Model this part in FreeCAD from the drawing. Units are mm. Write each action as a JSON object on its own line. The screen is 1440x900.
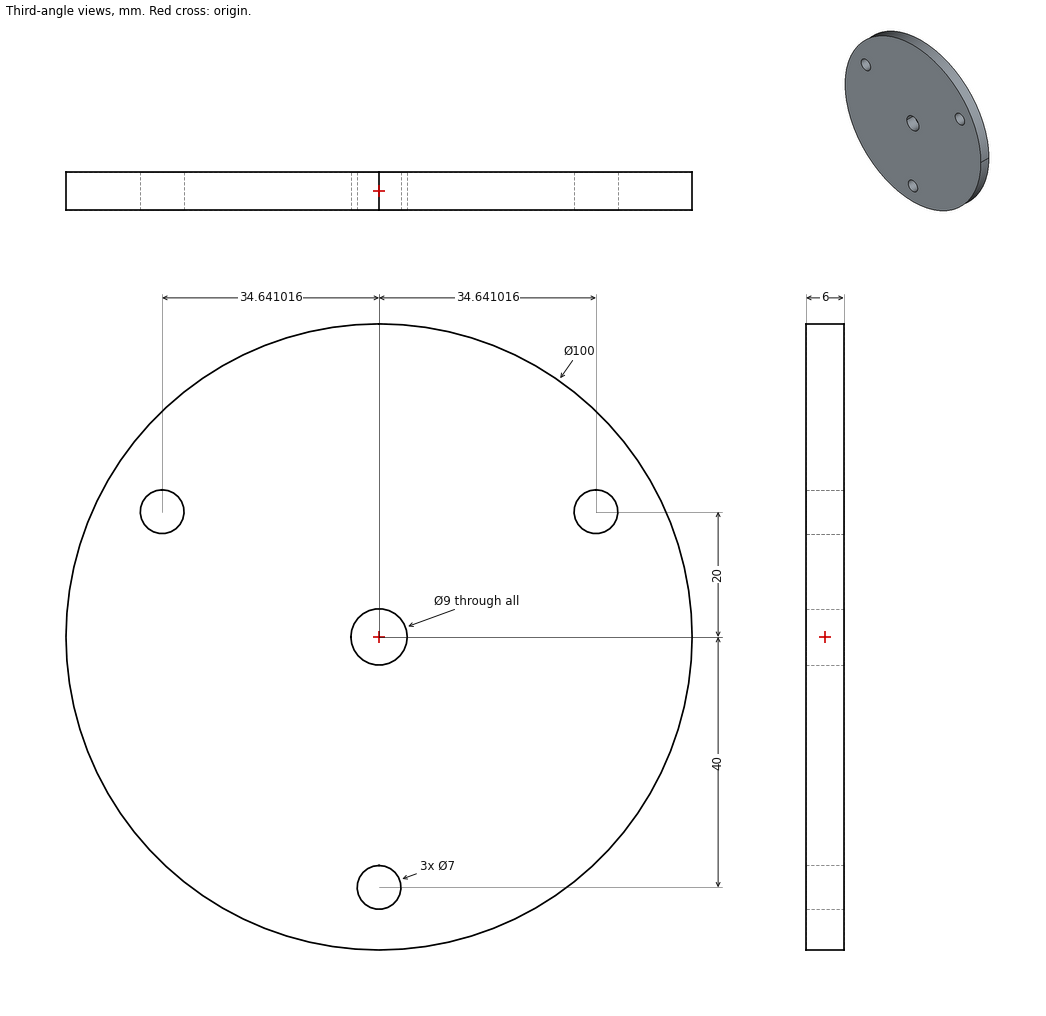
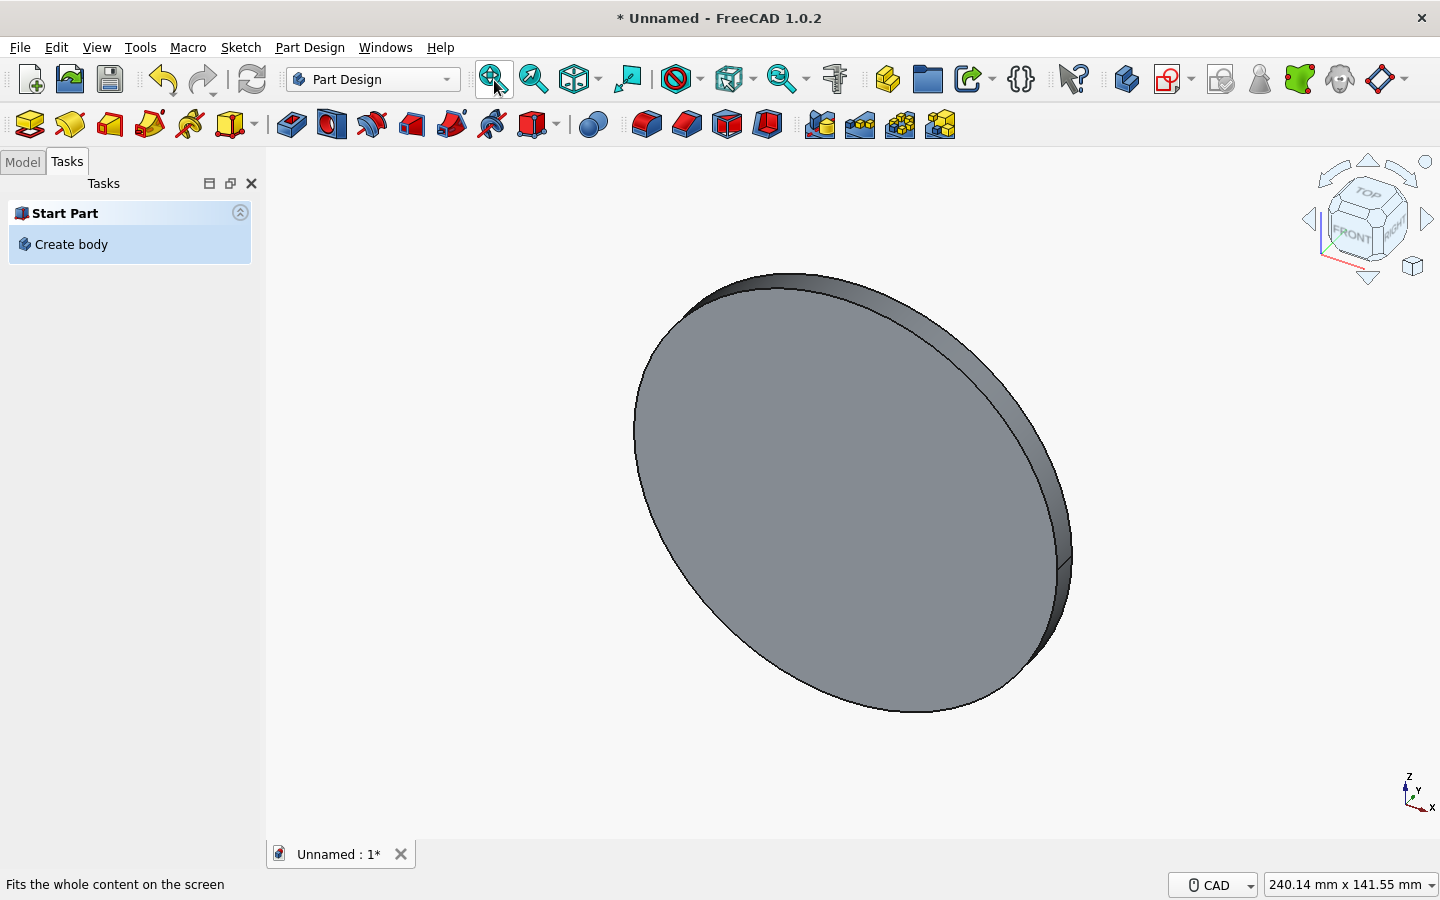
{"action": "key", "text": "4"}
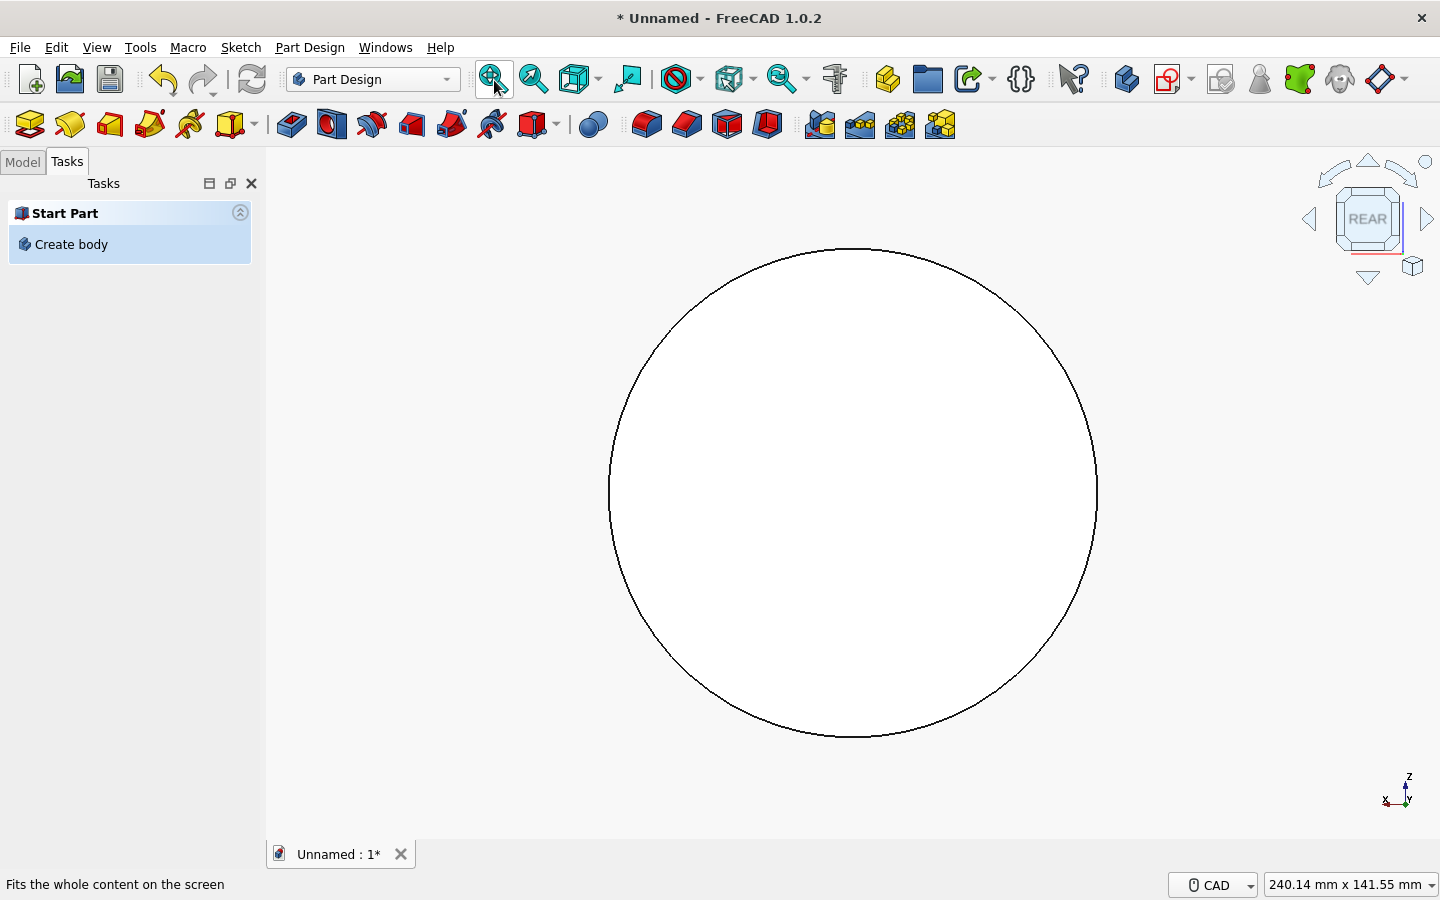
{"action": "left_click", "coordinate": [853, 492]}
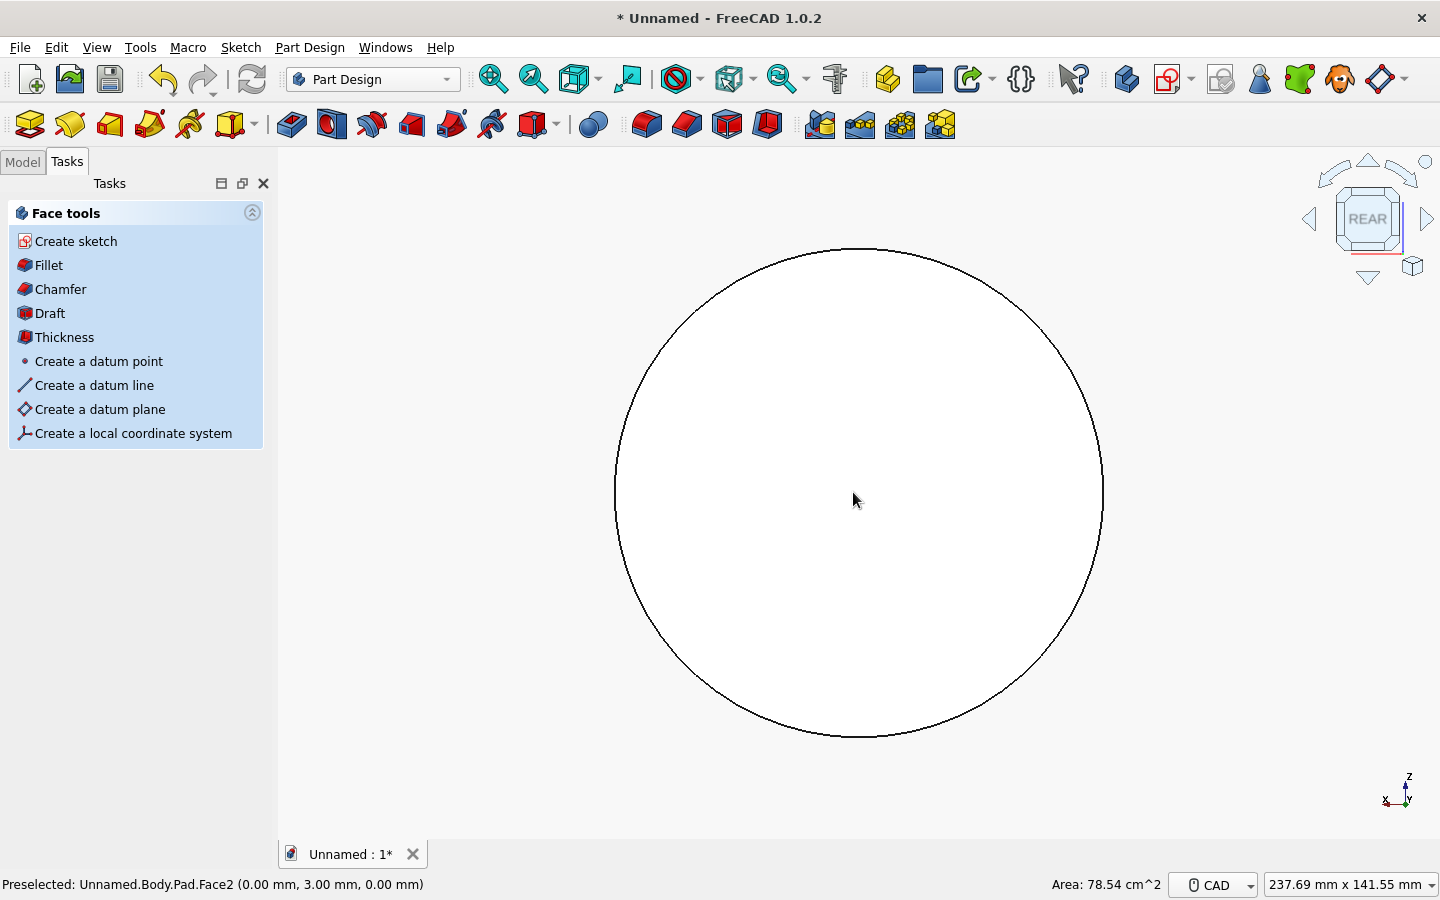
{"action": "left_click", "coordinate": [1168, 80]}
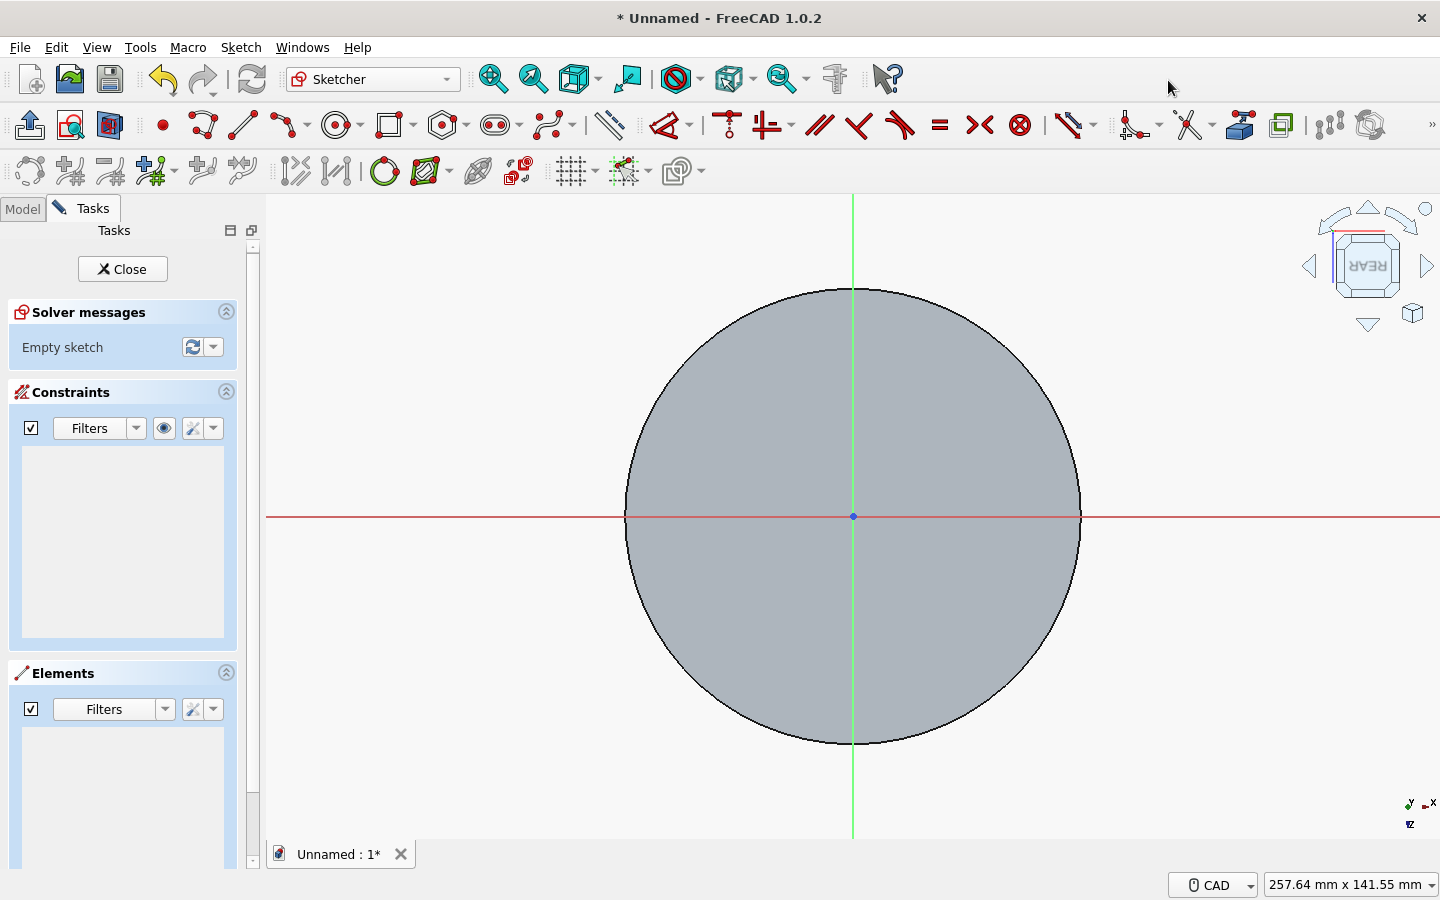
{"action": "scroll", "coordinate": [992, 378], "scroll_direction": "up", "scroll_amount": 2}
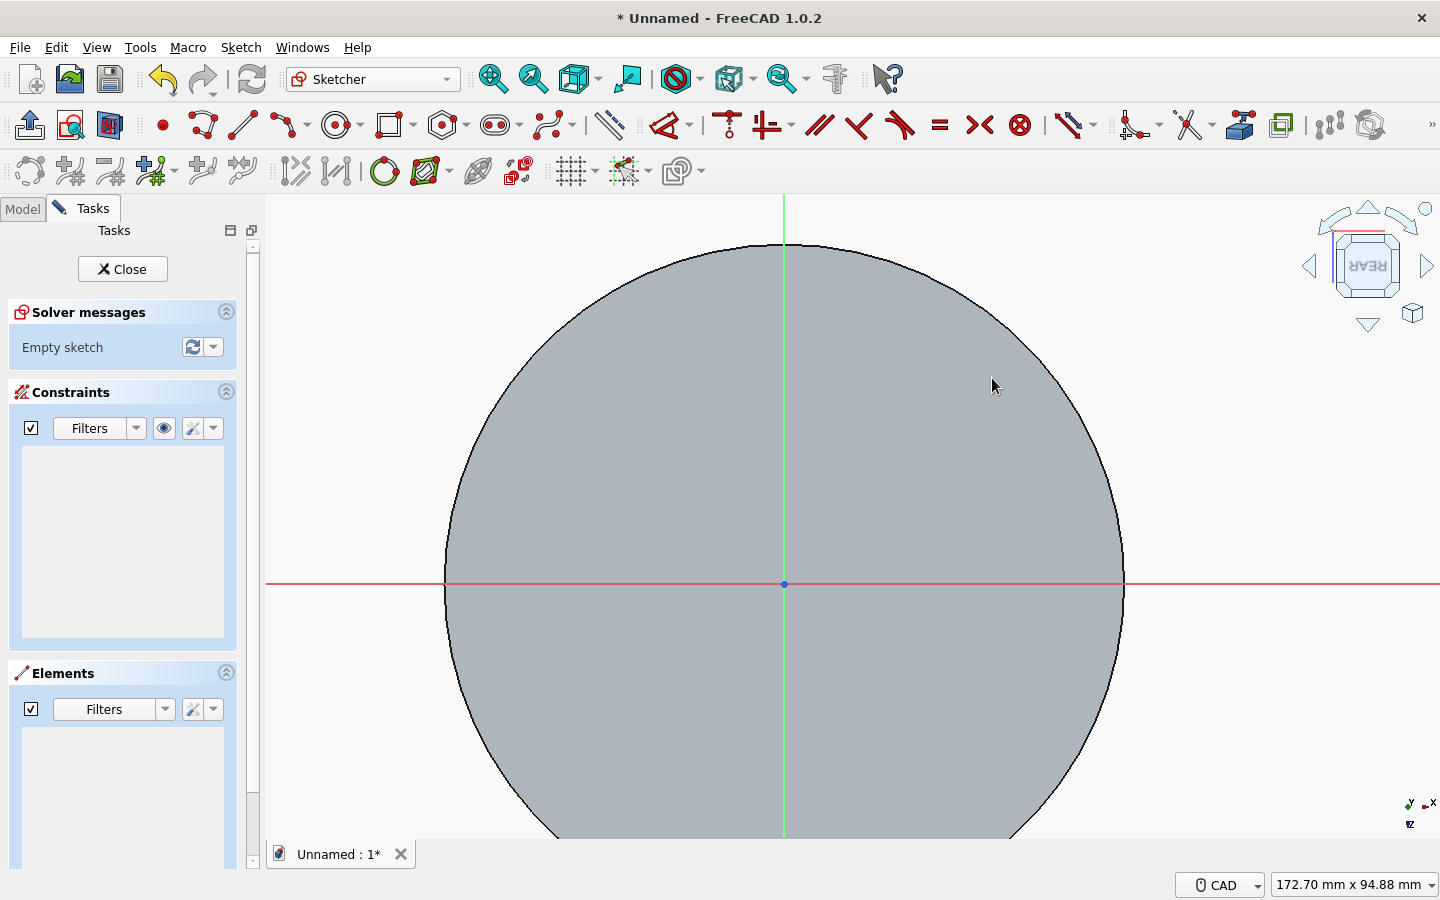
{"action": "left_click", "coordinate": [336, 126]}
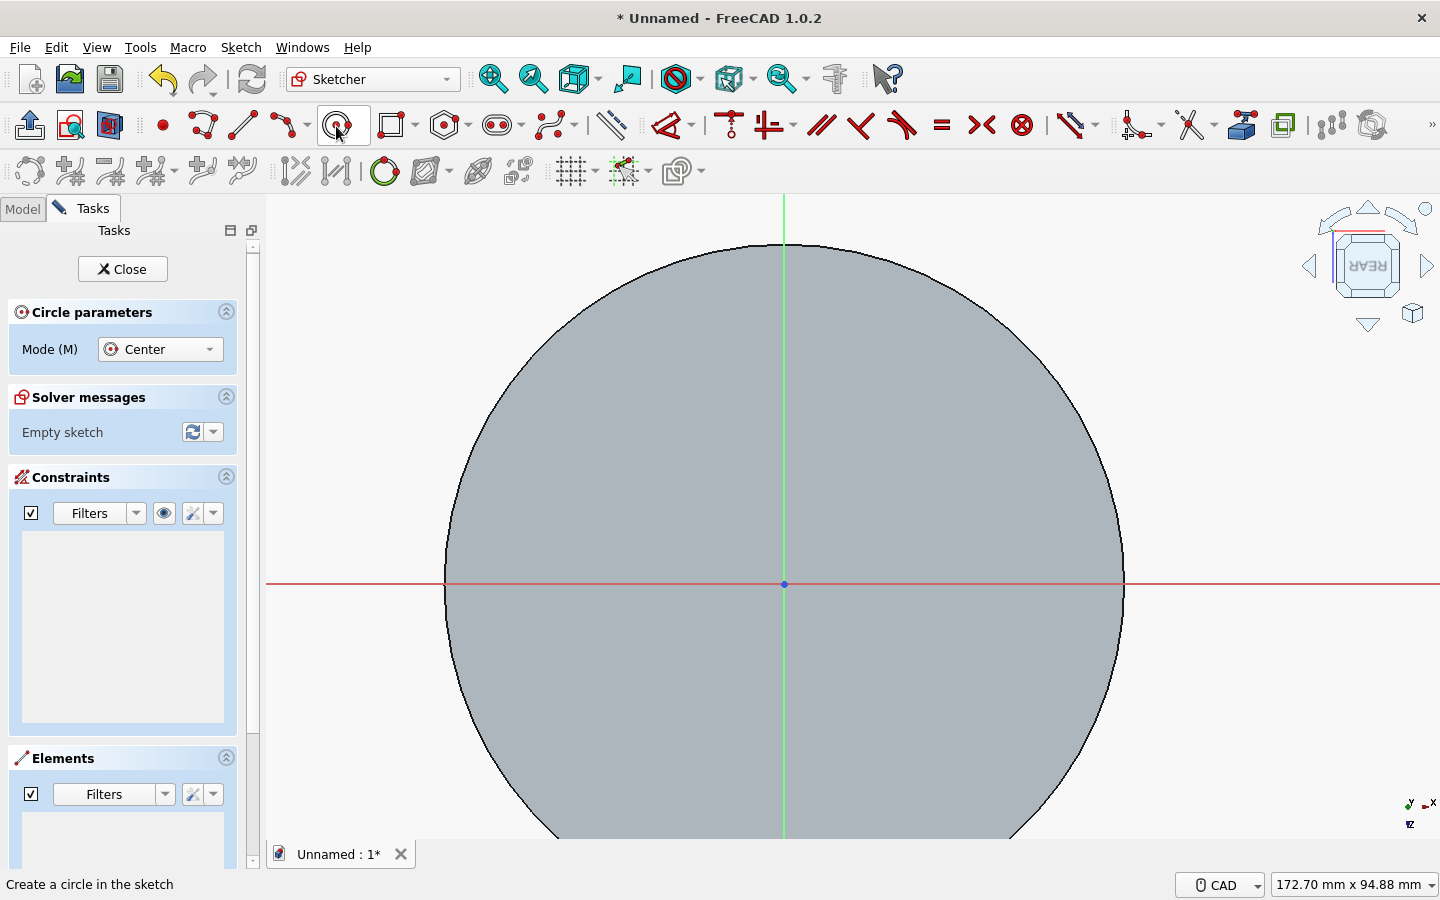
{"action": "left_click", "coordinate": [784, 313]}
{"action": "mouse_move", "coordinate": [801, 296]}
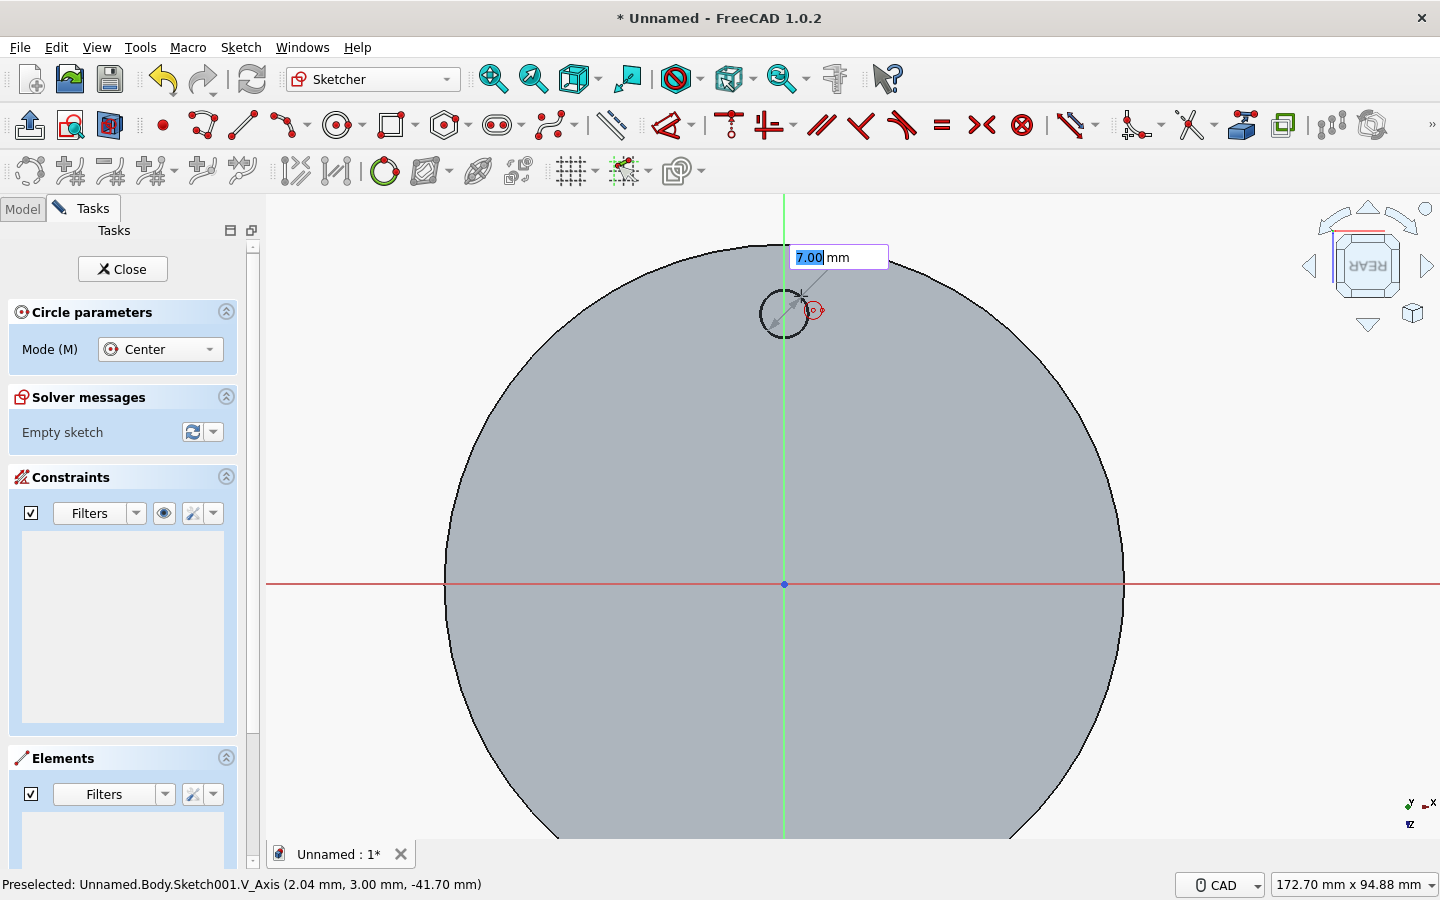
{"action": "type", "text": "7"}
{"action": "key", "text": "Return"}